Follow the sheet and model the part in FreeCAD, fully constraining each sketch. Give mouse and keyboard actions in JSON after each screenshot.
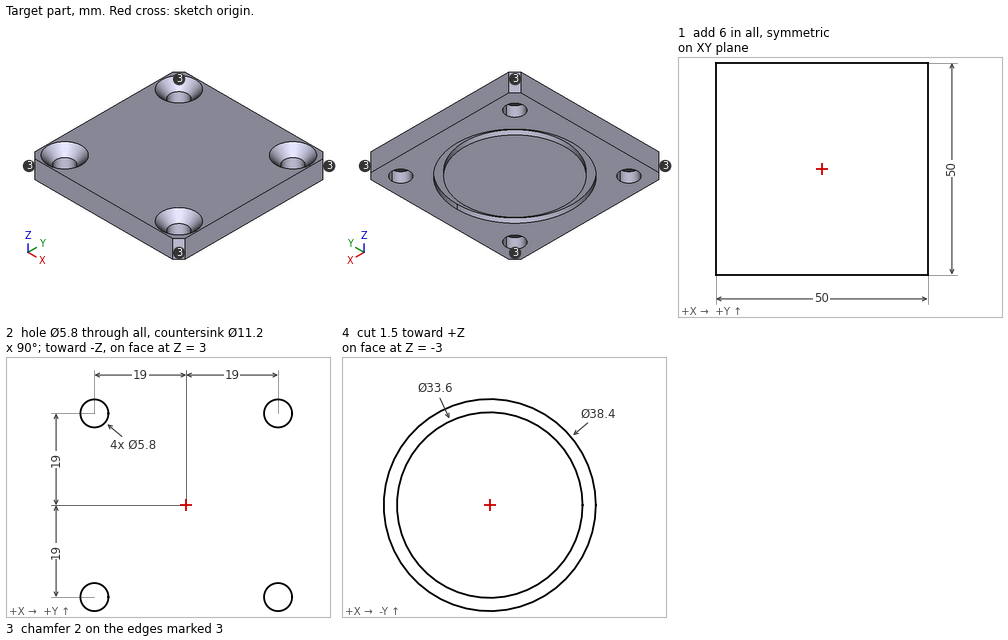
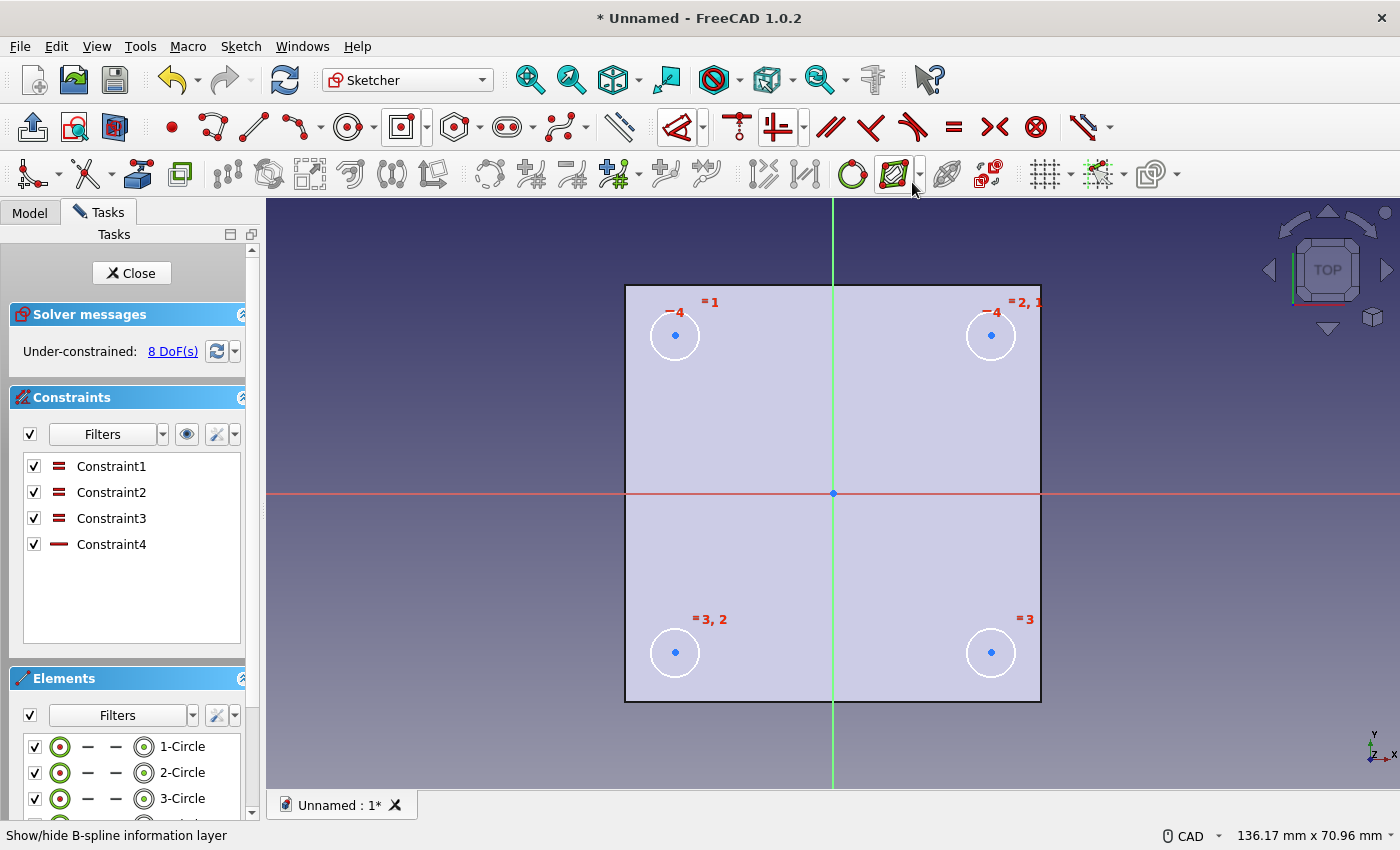
{"action": "left_click", "coordinate": [675, 336]}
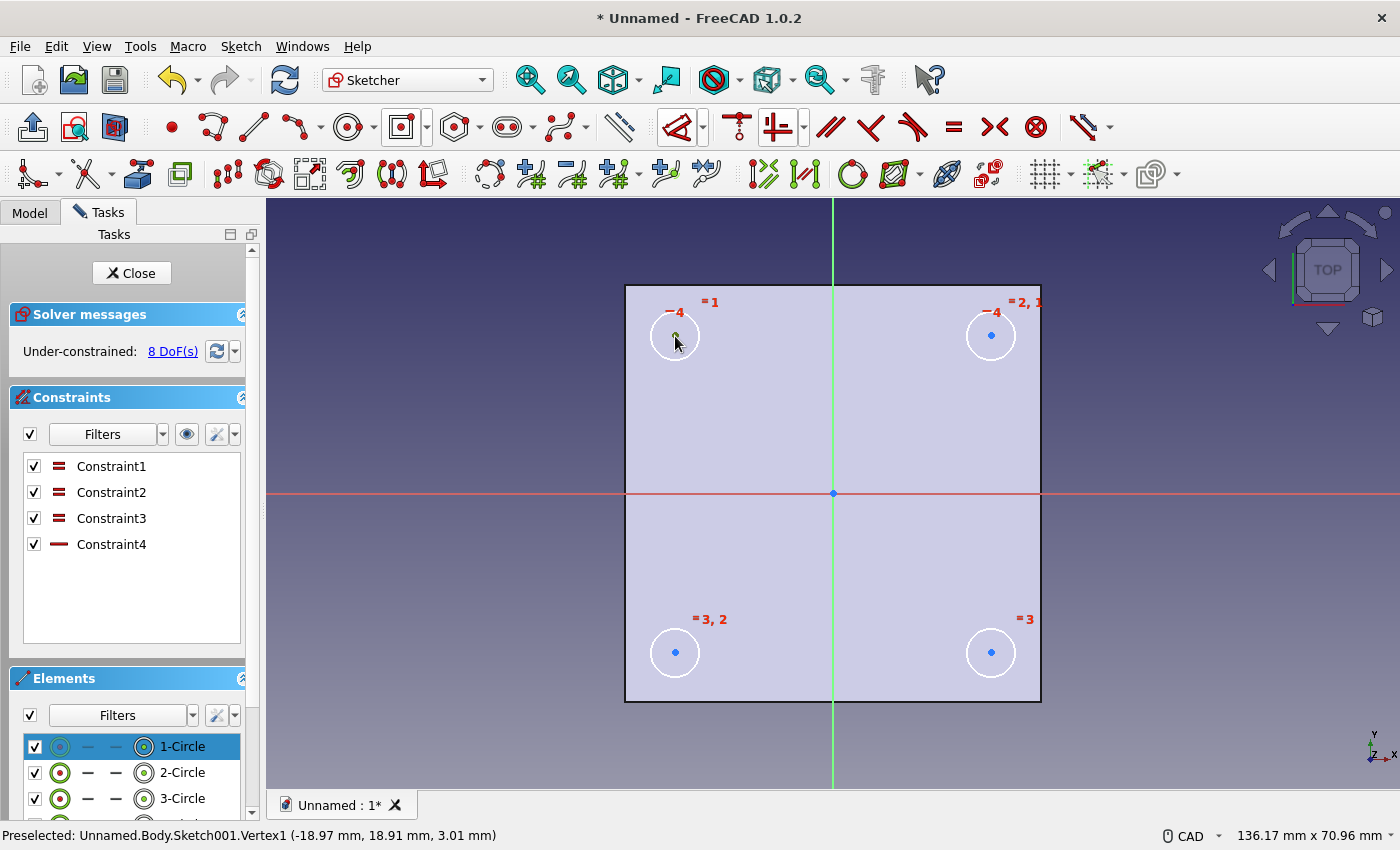
{"action": "left_click", "coordinate": [675, 653]}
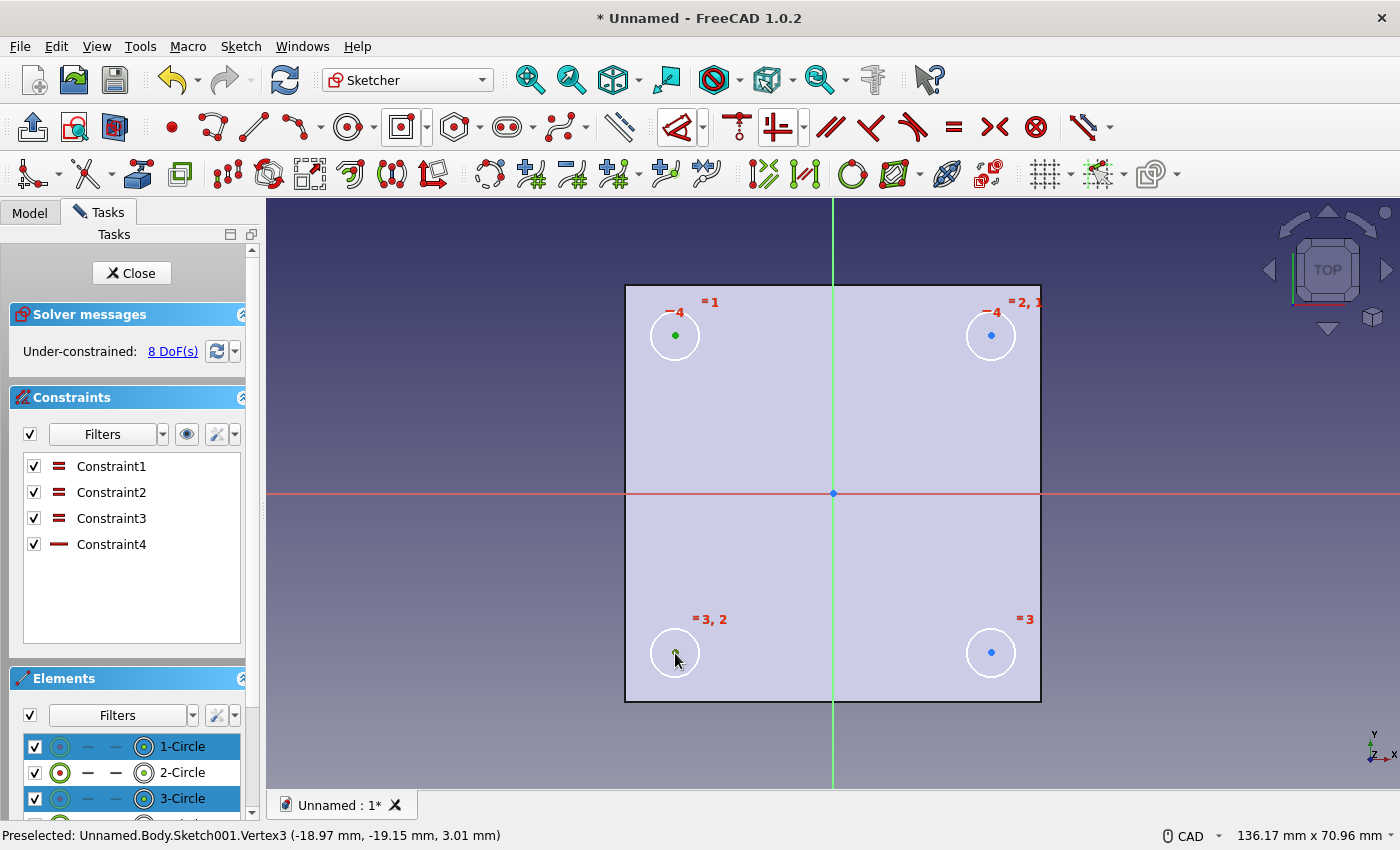
{"action": "left_click", "coordinate": [804, 128]}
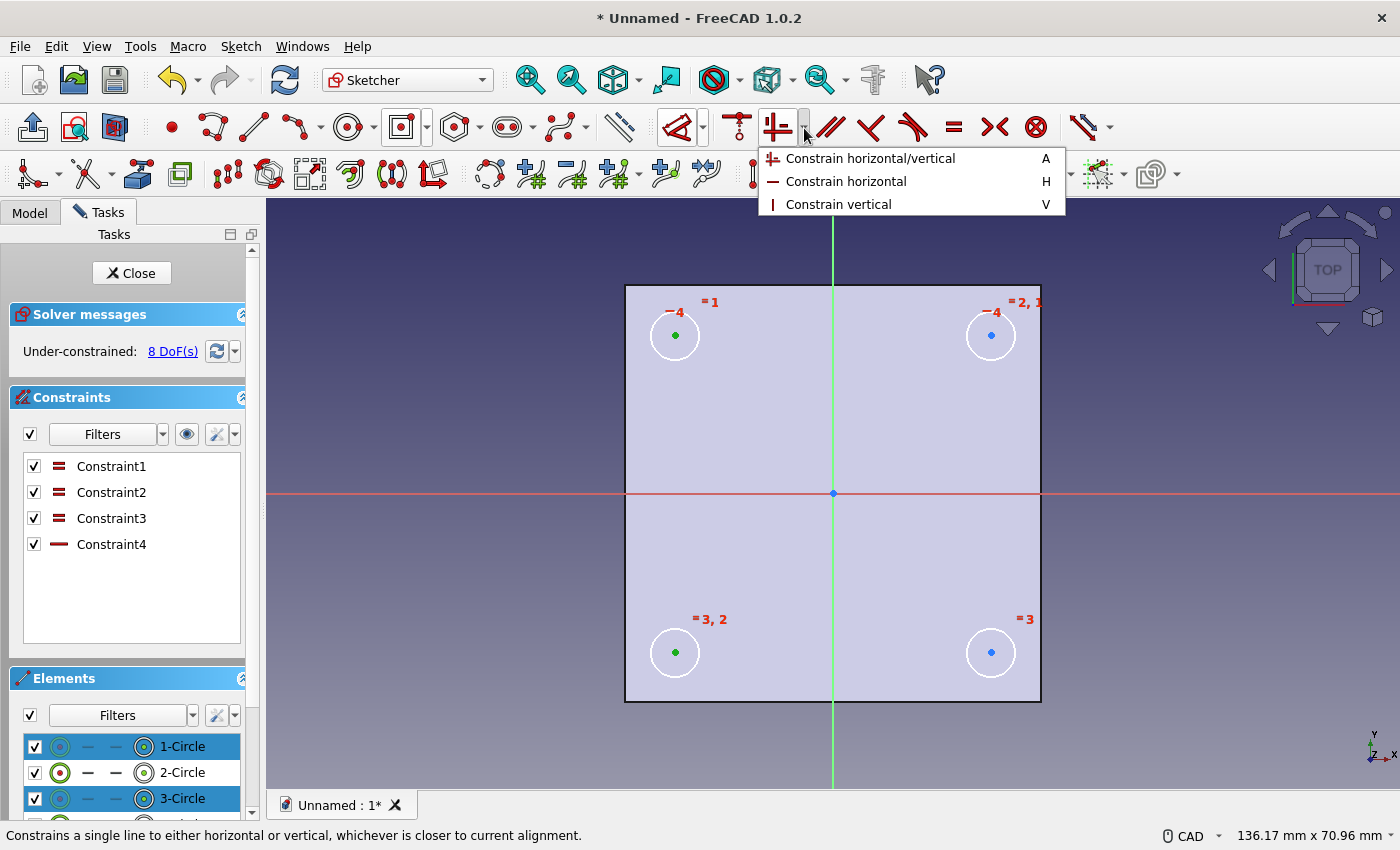
{"action": "left_click", "coordinate": [912, 204]}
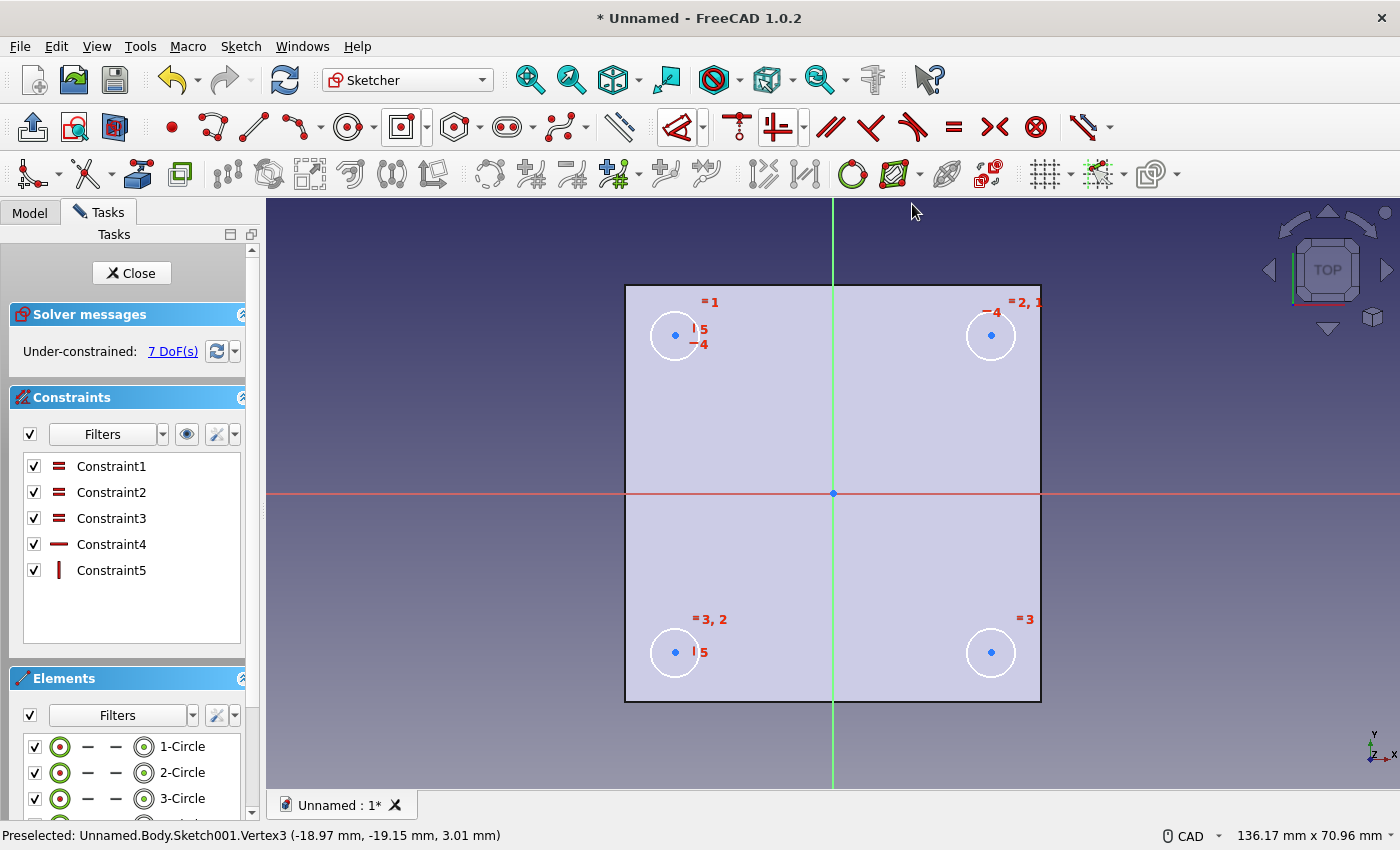
{"action": "left_click", "coordinate": [991, 336]}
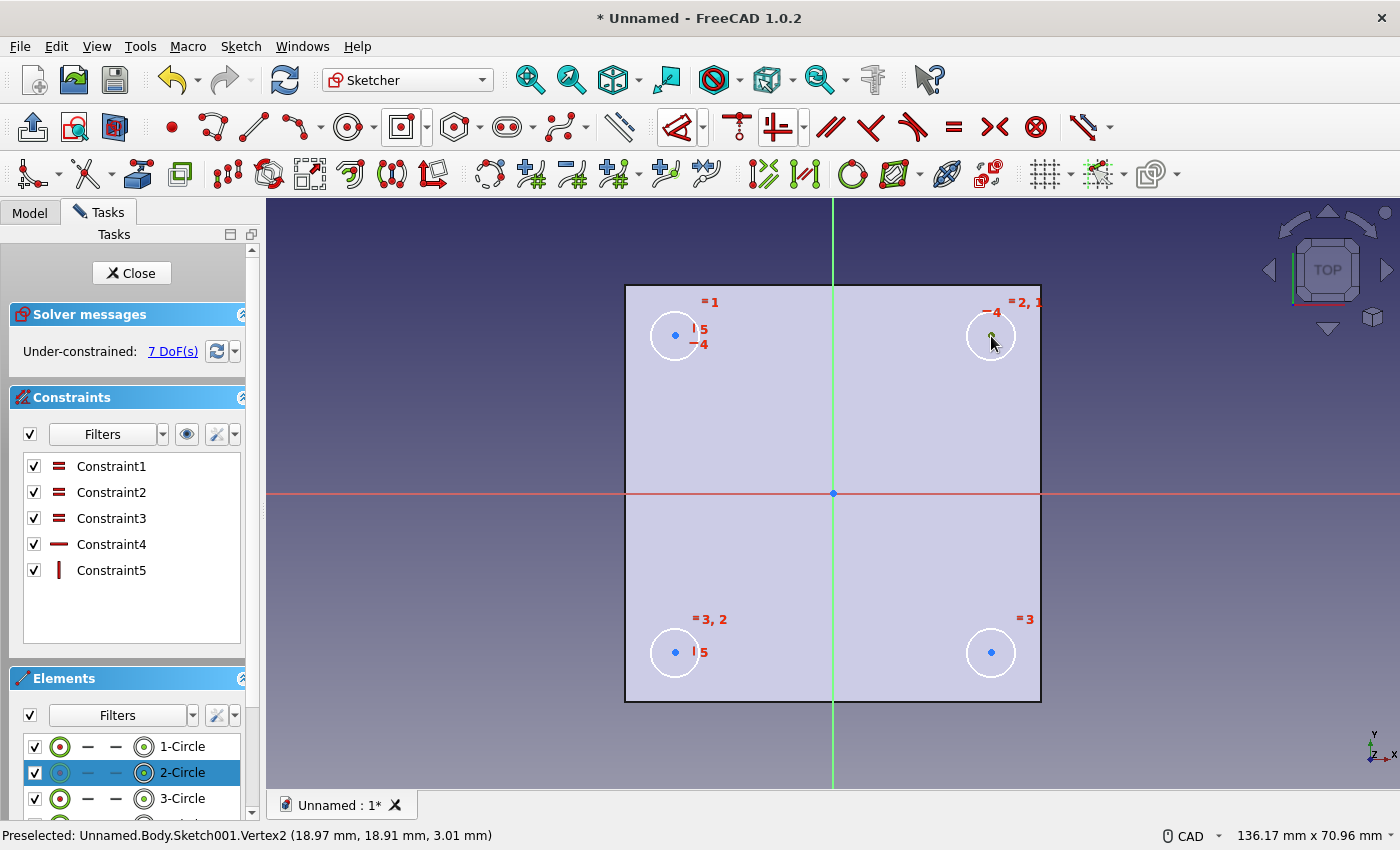
{"action": "left_click", "coordinate": [991, 653]}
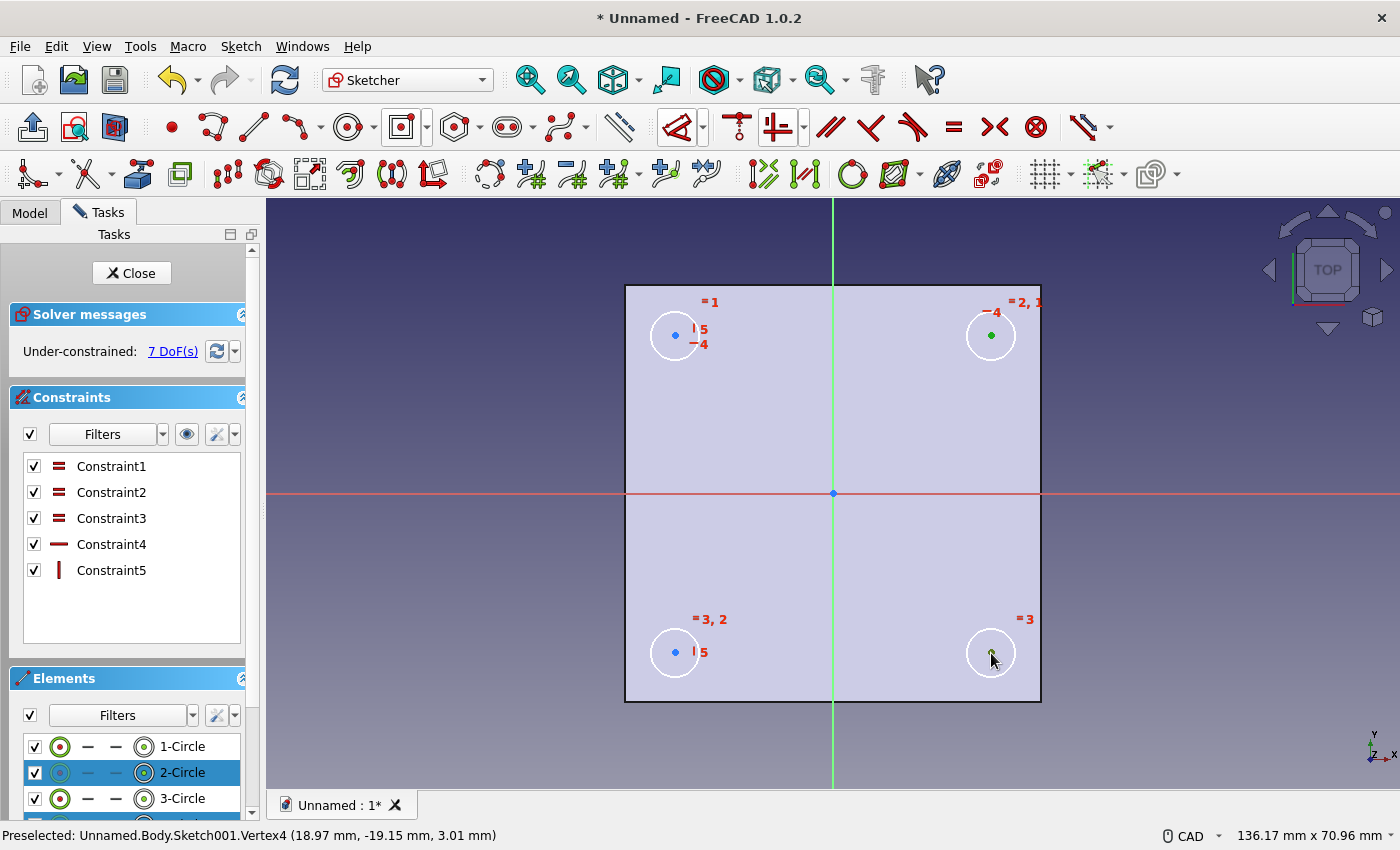
{"action": "key", "text": "v"}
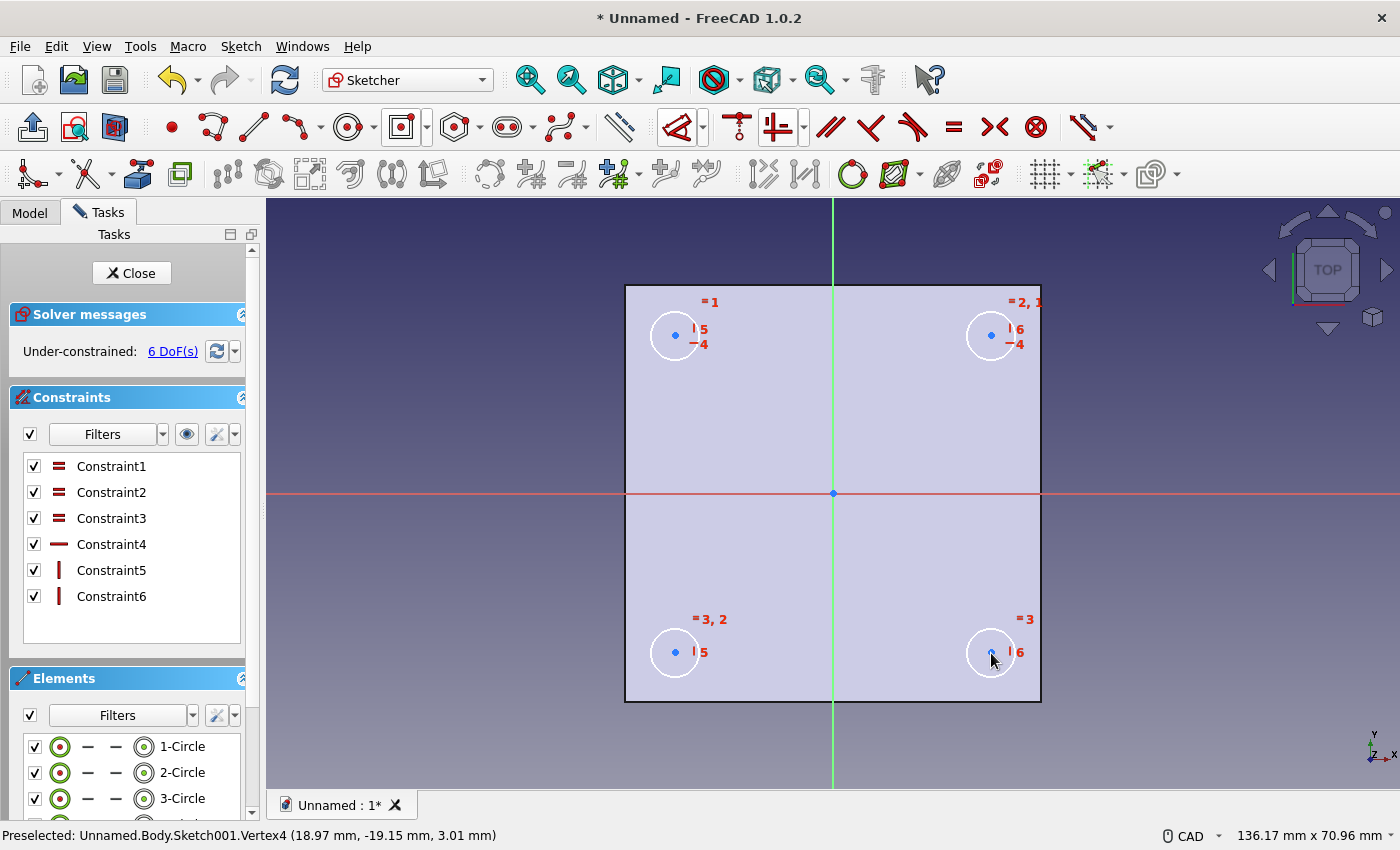
{"action": "left_click", "coordinate": [675, 653]}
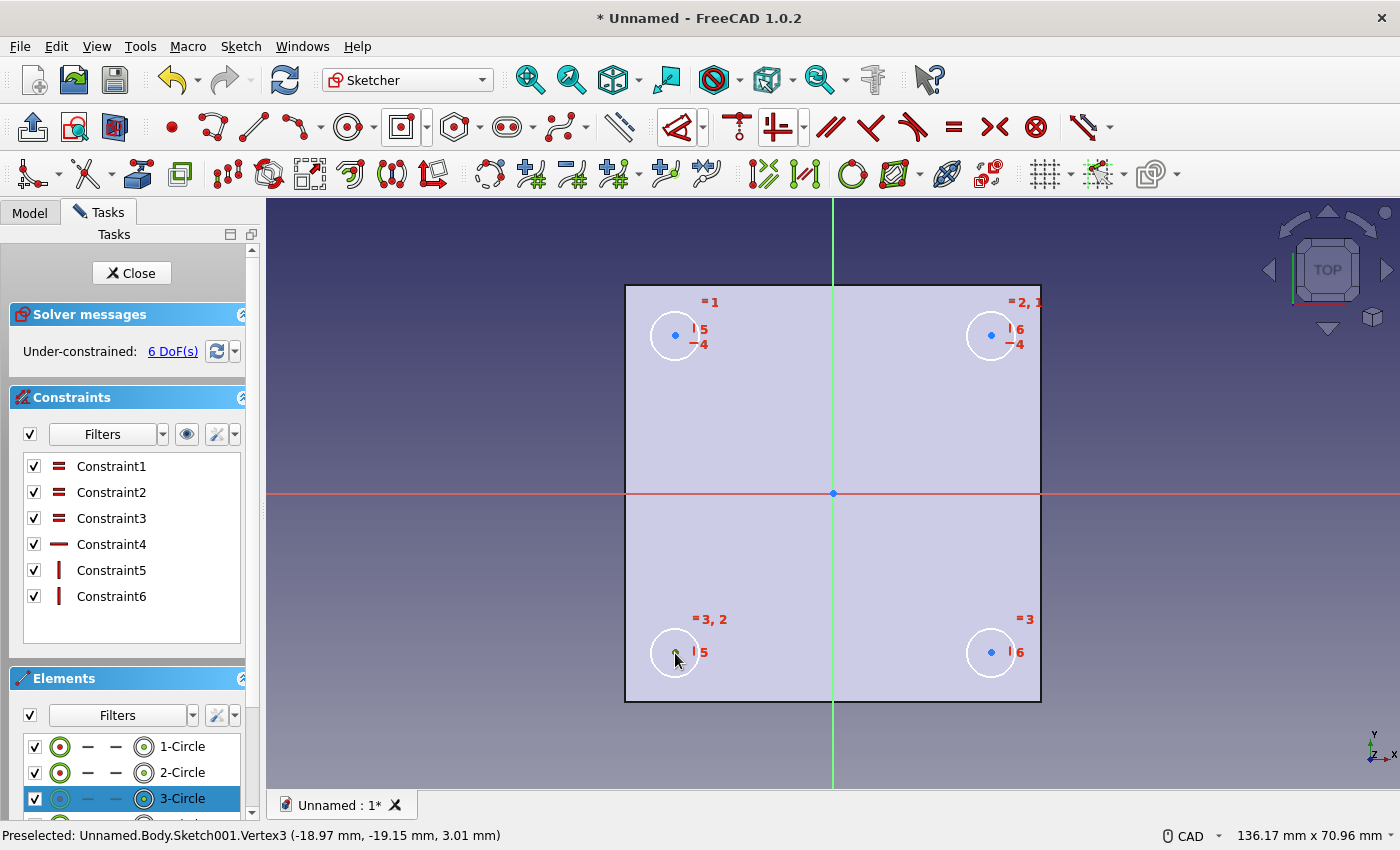
{"action": "left_click", "coordinate": [991, 653]}